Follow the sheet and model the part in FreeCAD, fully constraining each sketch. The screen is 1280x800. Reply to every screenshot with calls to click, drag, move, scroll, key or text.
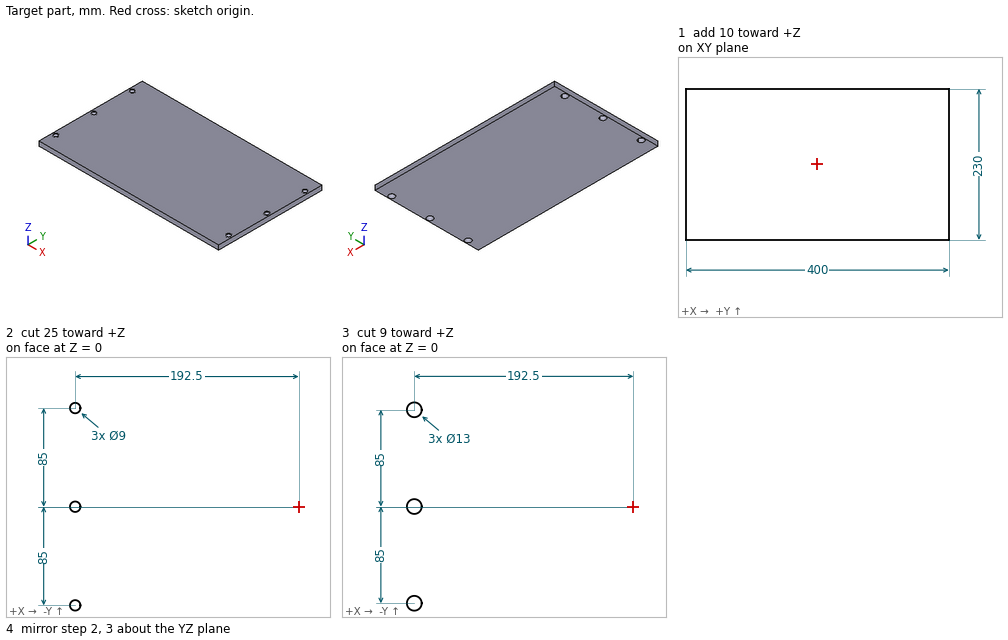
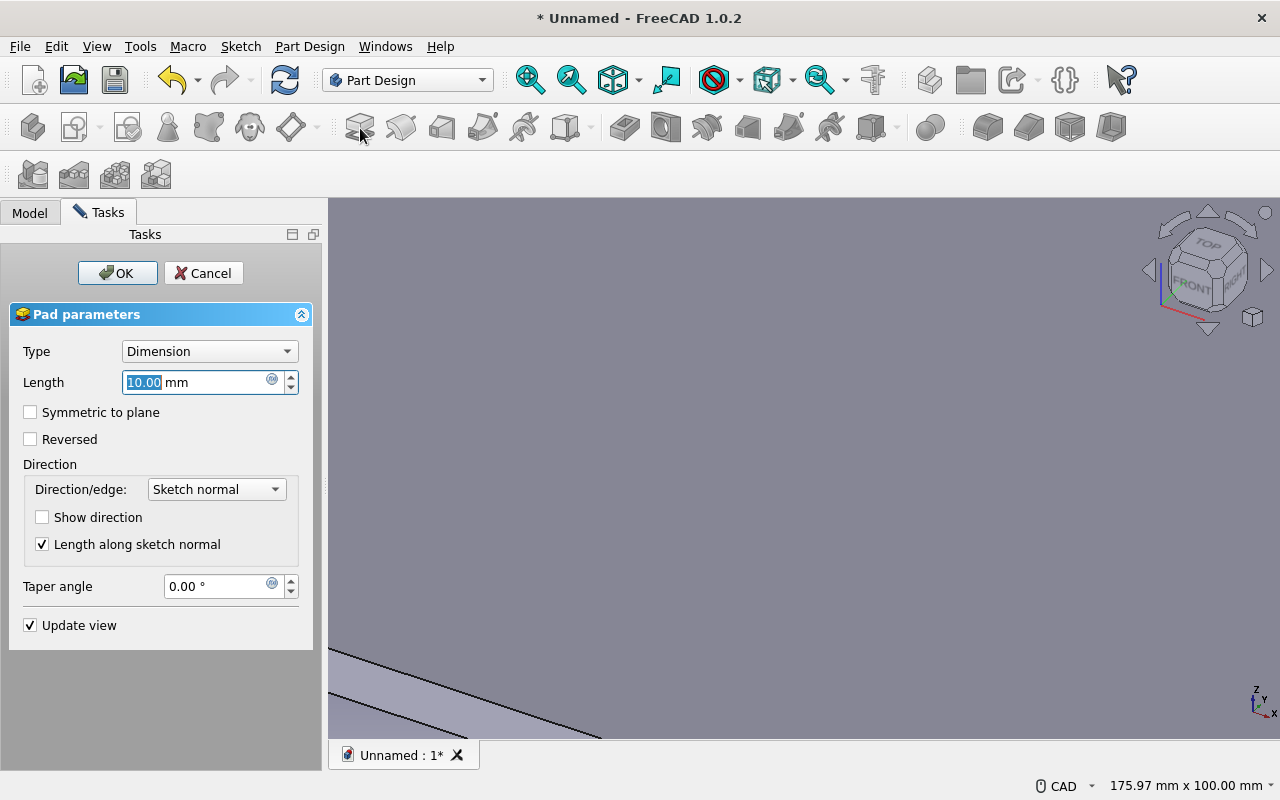
text(10)
key(Tab)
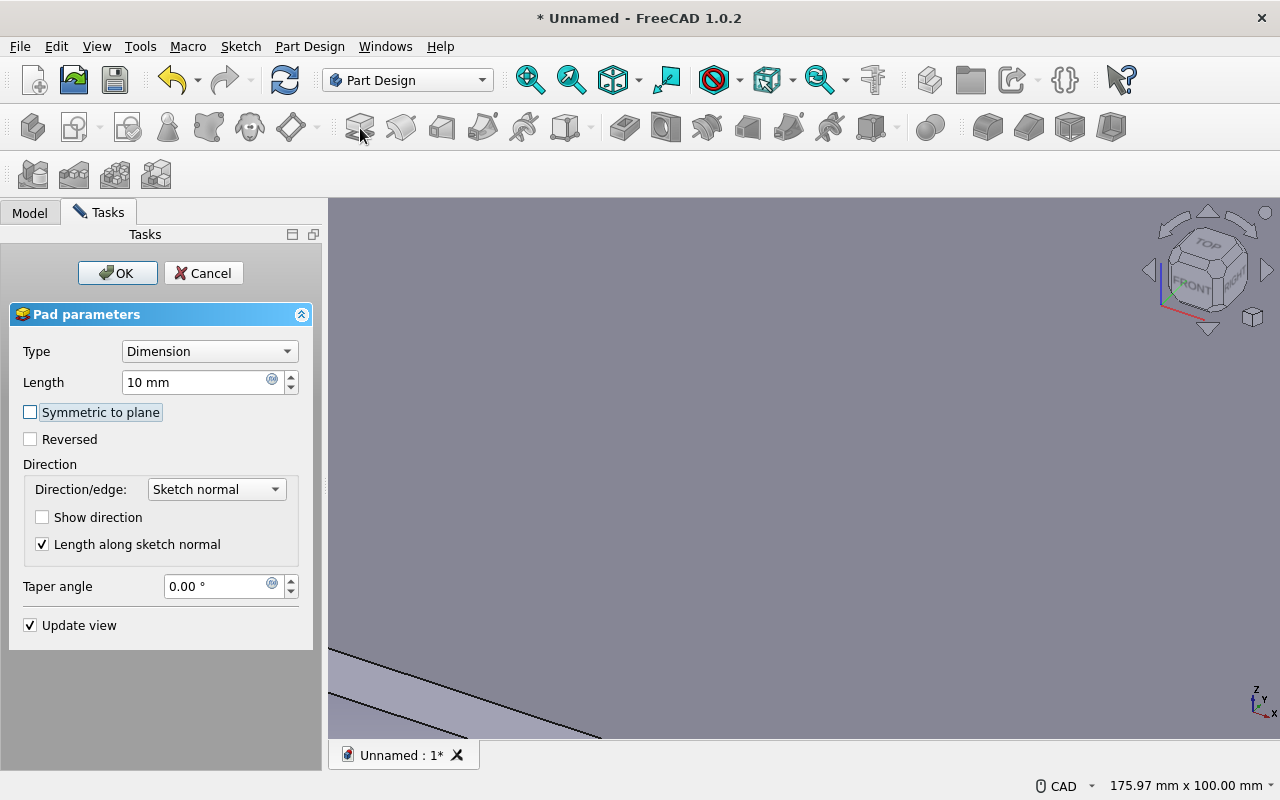
click(118, 273)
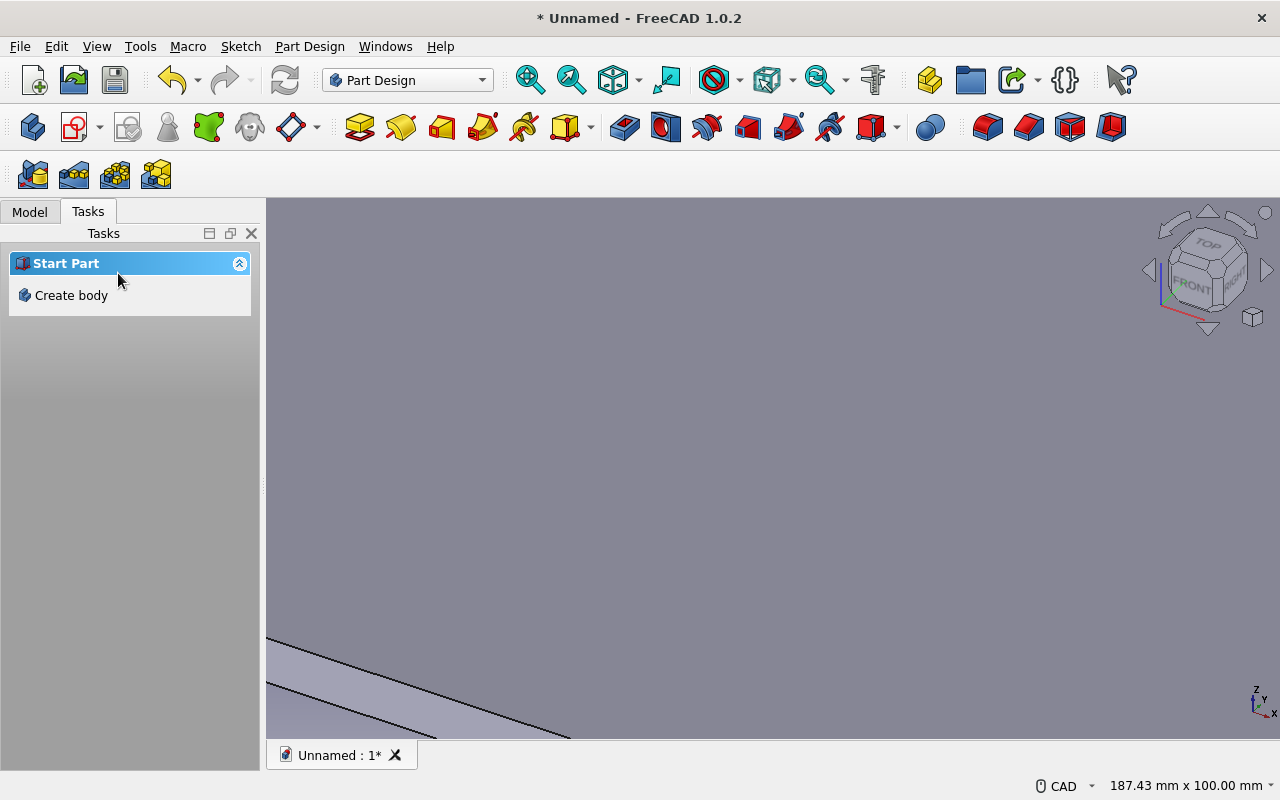
click(531, 80)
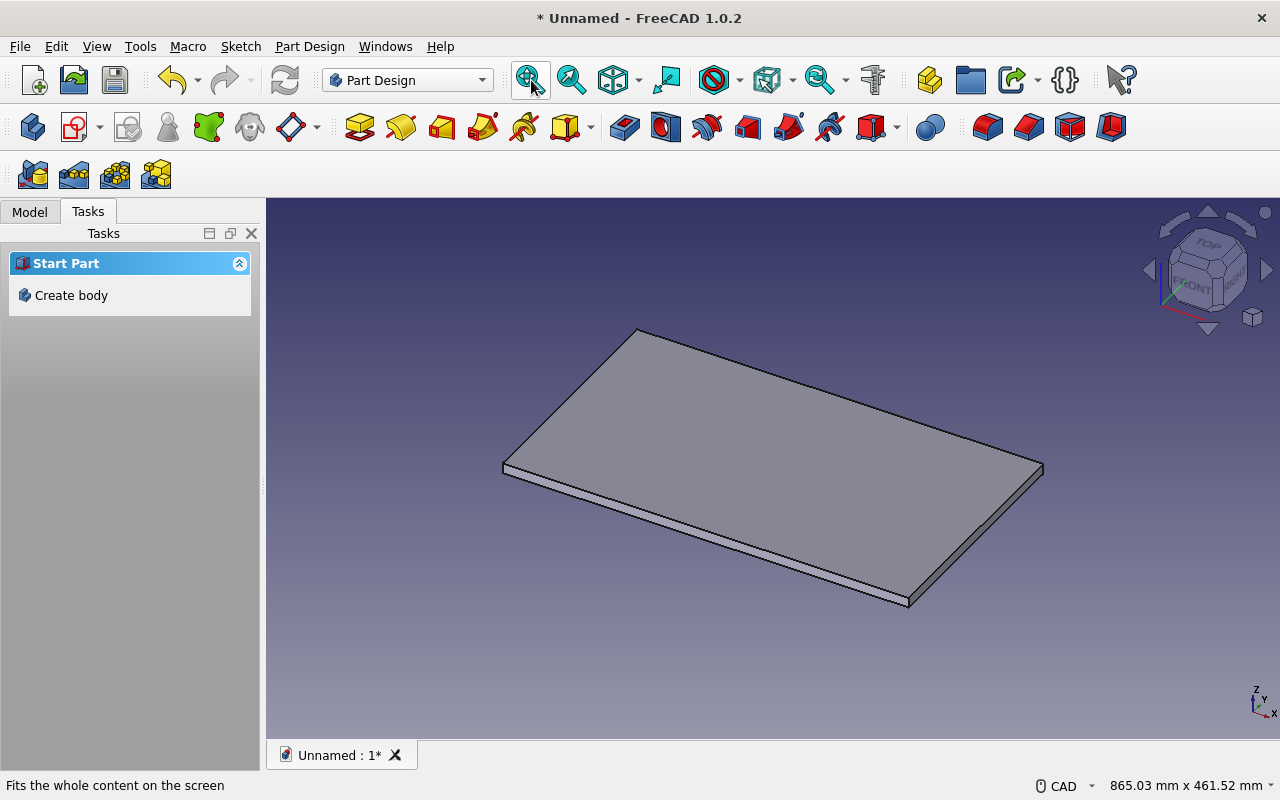
key(5)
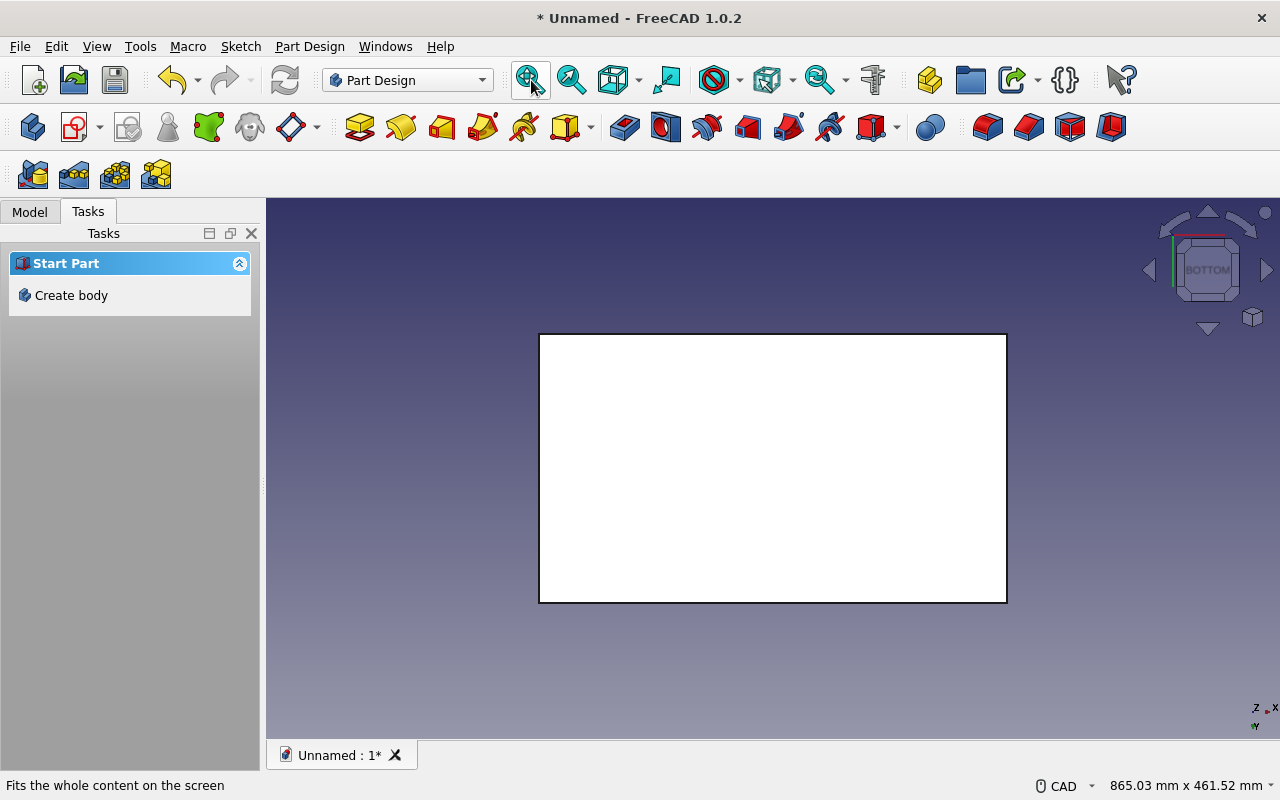
click(840, 467)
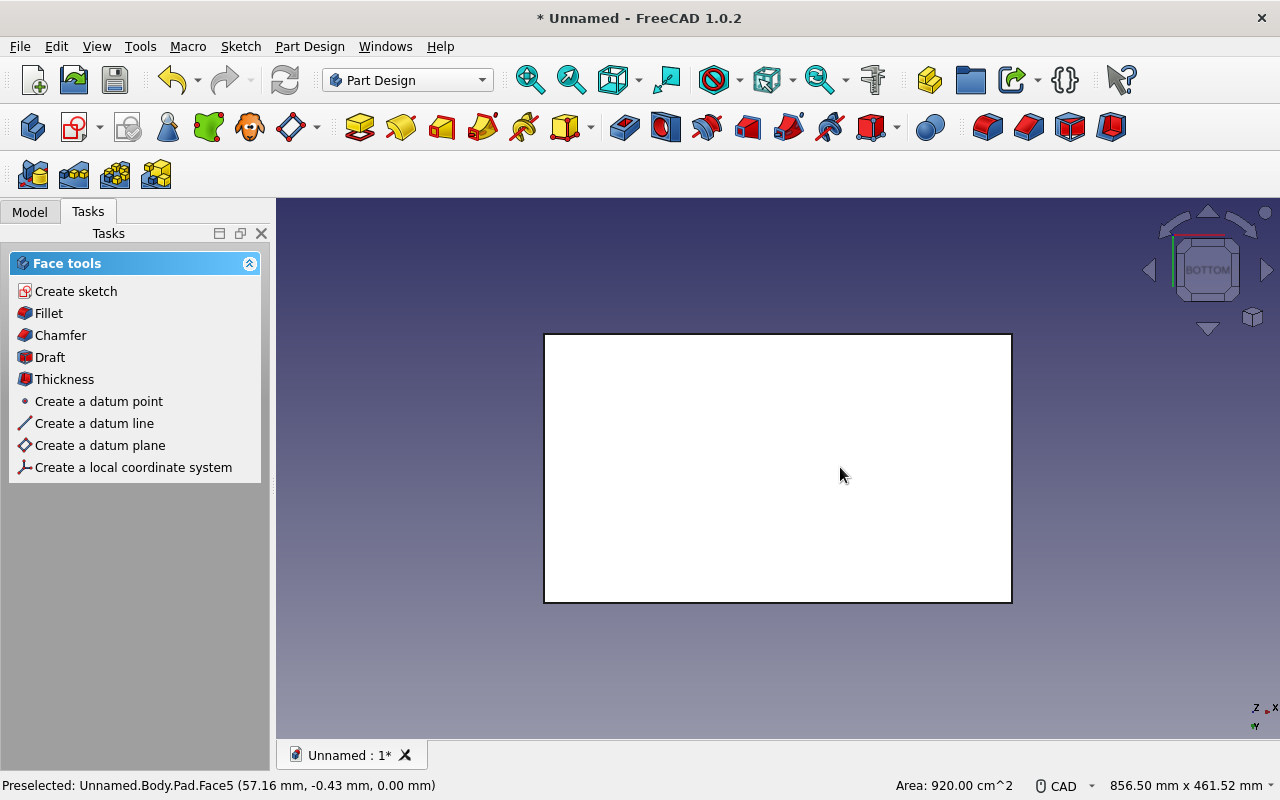
click(74, 128)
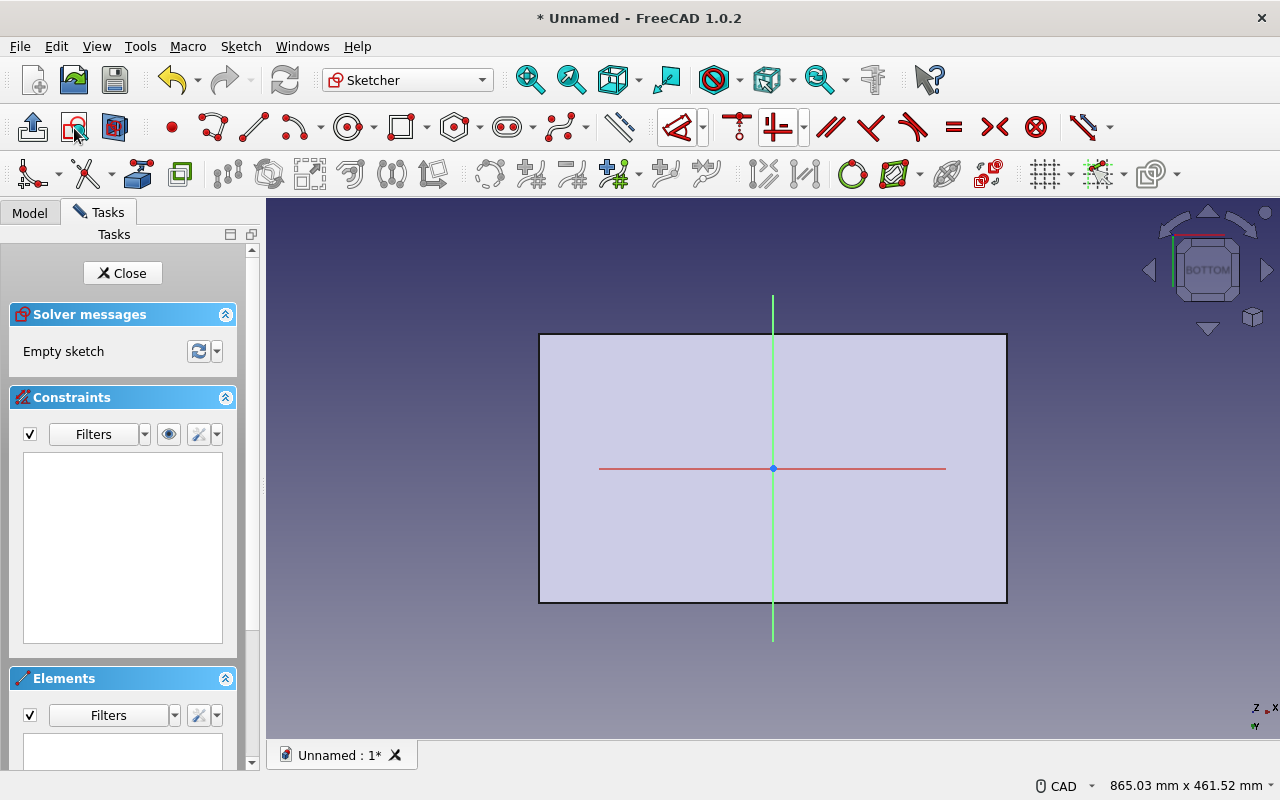
scroll(562, 469, up, 2)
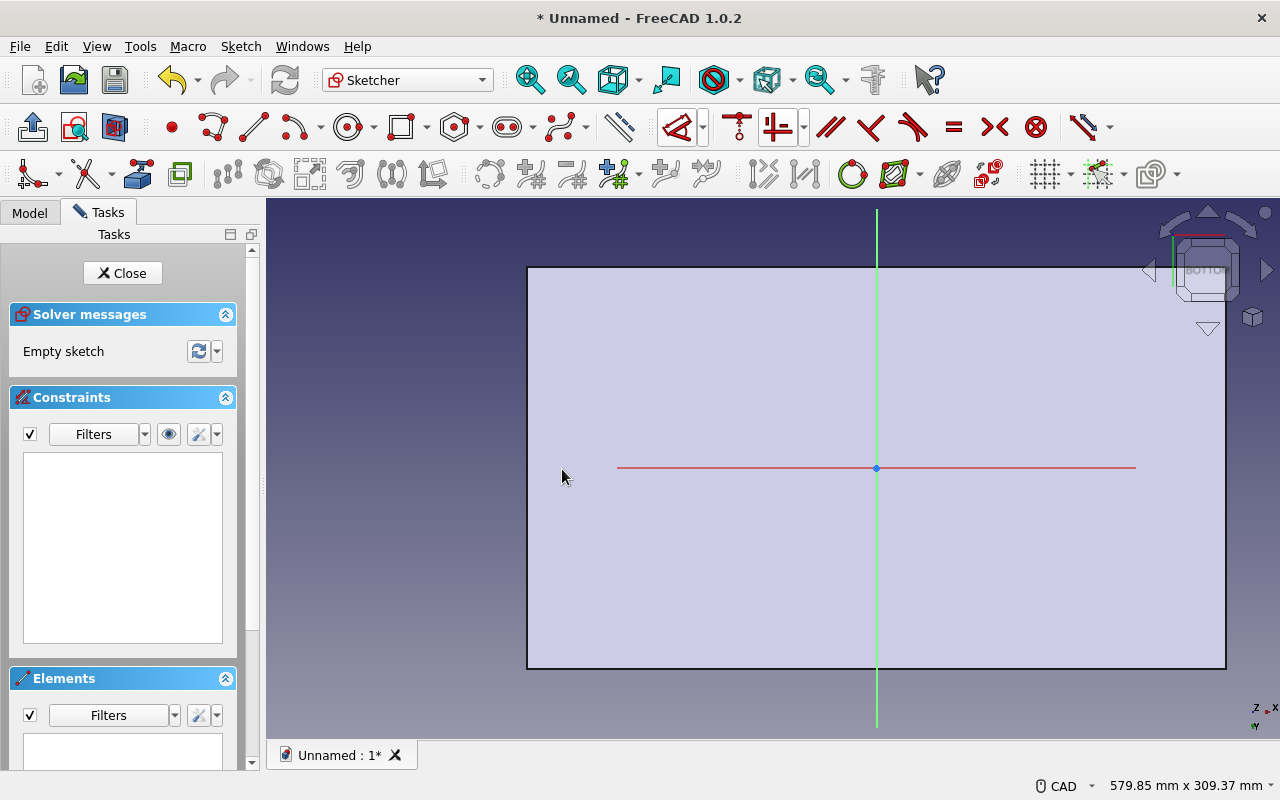
click(348, 128)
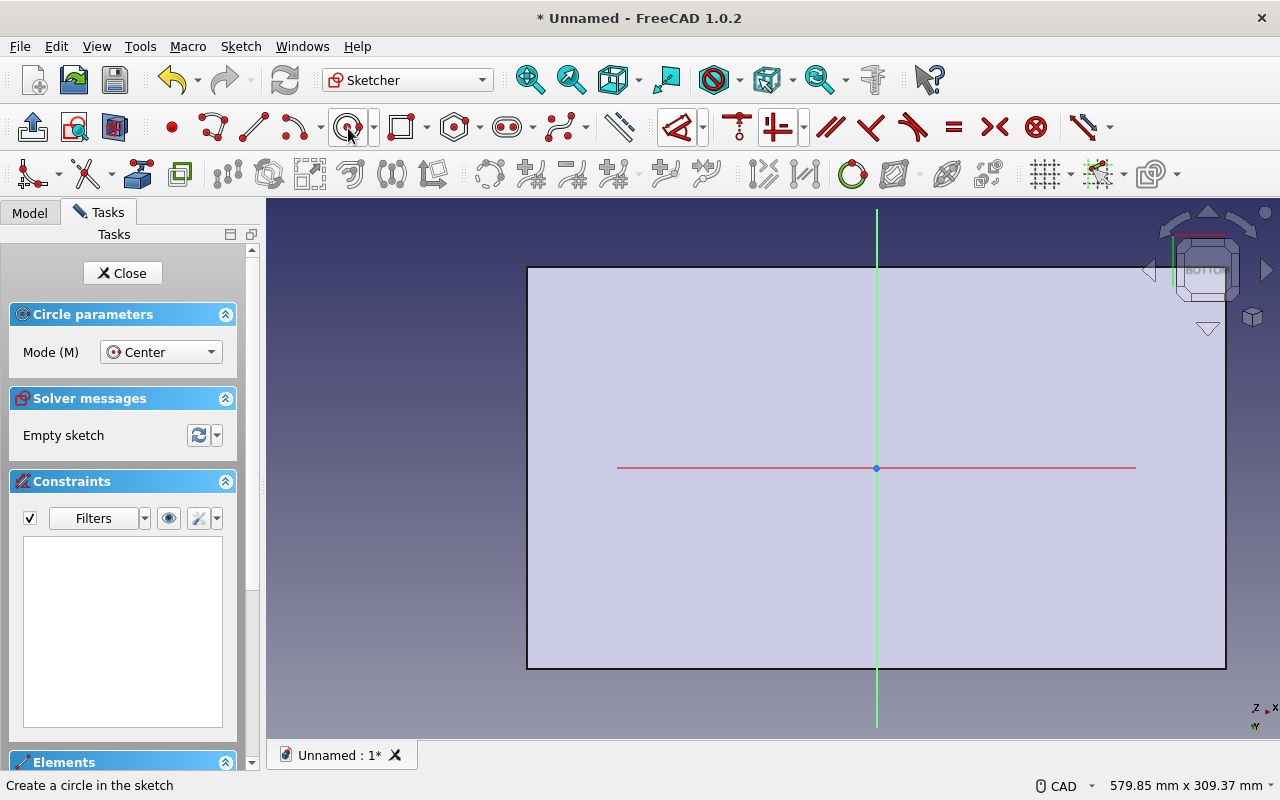
scroll(540, 319, up, 6)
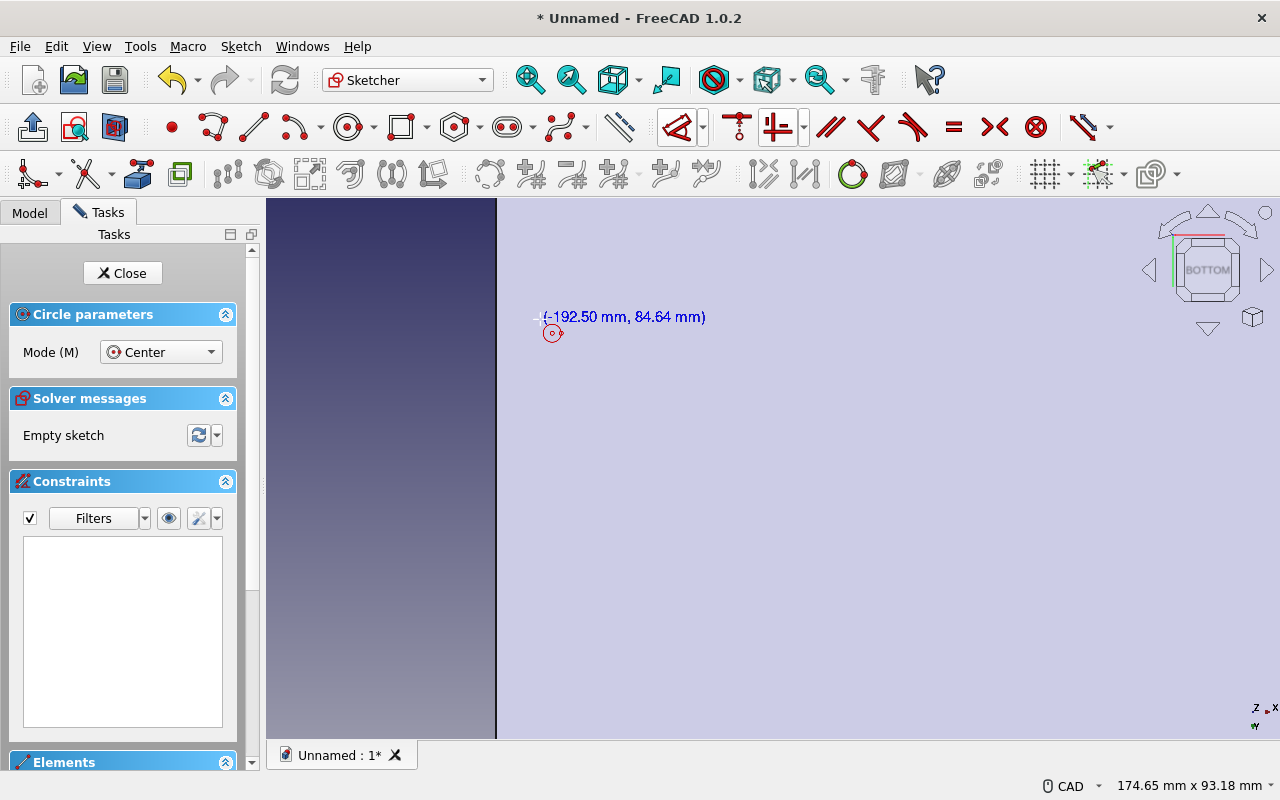
click(539, 320)
move(558, 301)